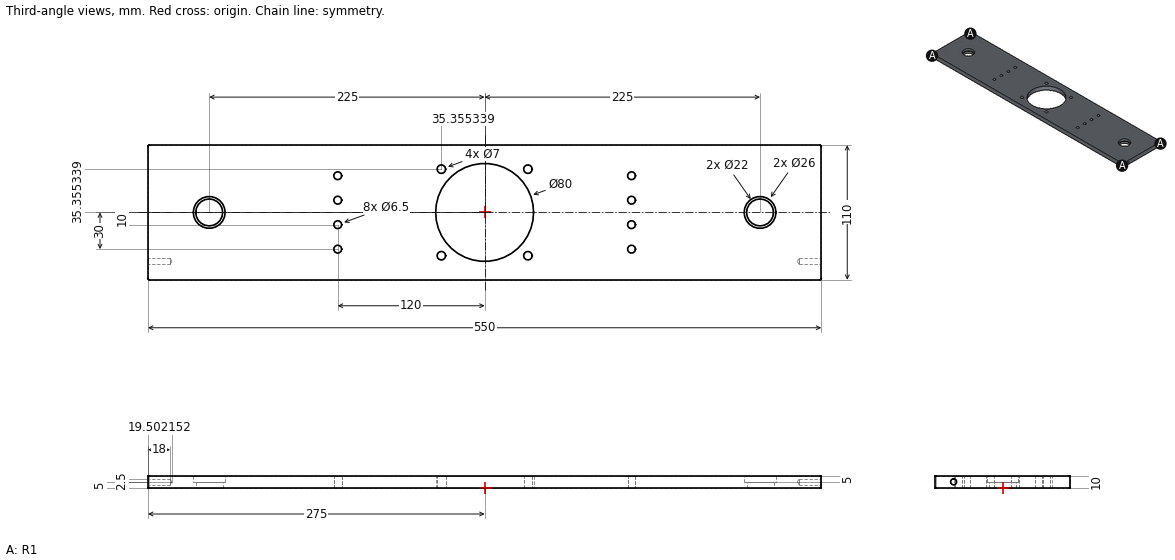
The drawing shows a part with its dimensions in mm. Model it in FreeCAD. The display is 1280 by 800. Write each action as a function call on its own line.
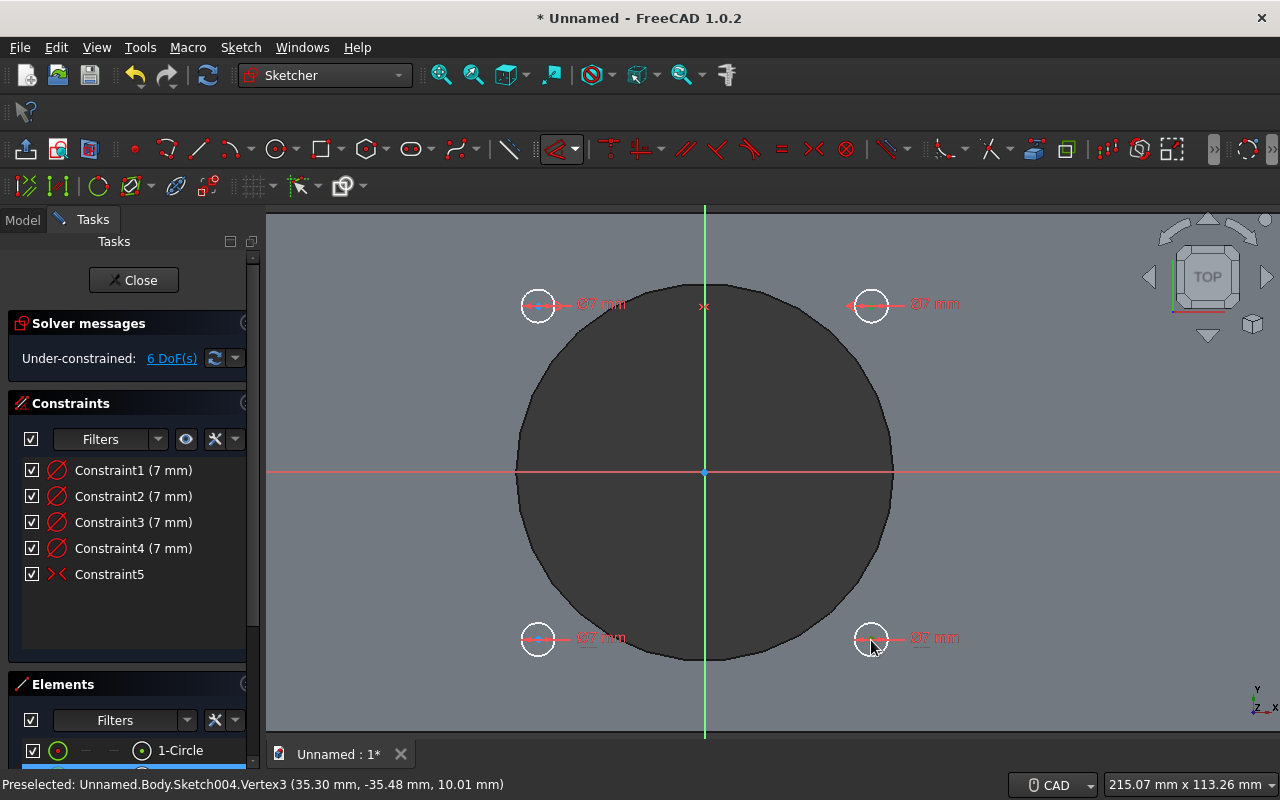
click(353, 472)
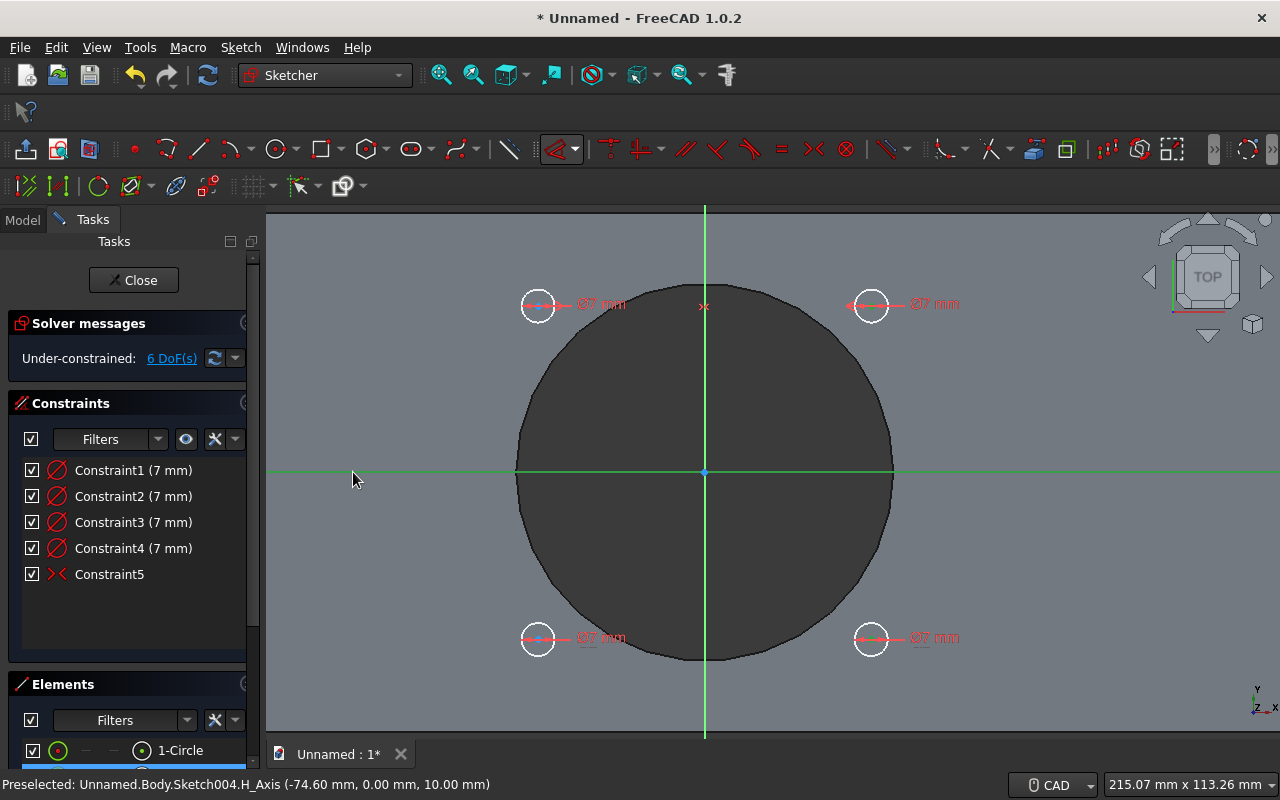
click(814, 150)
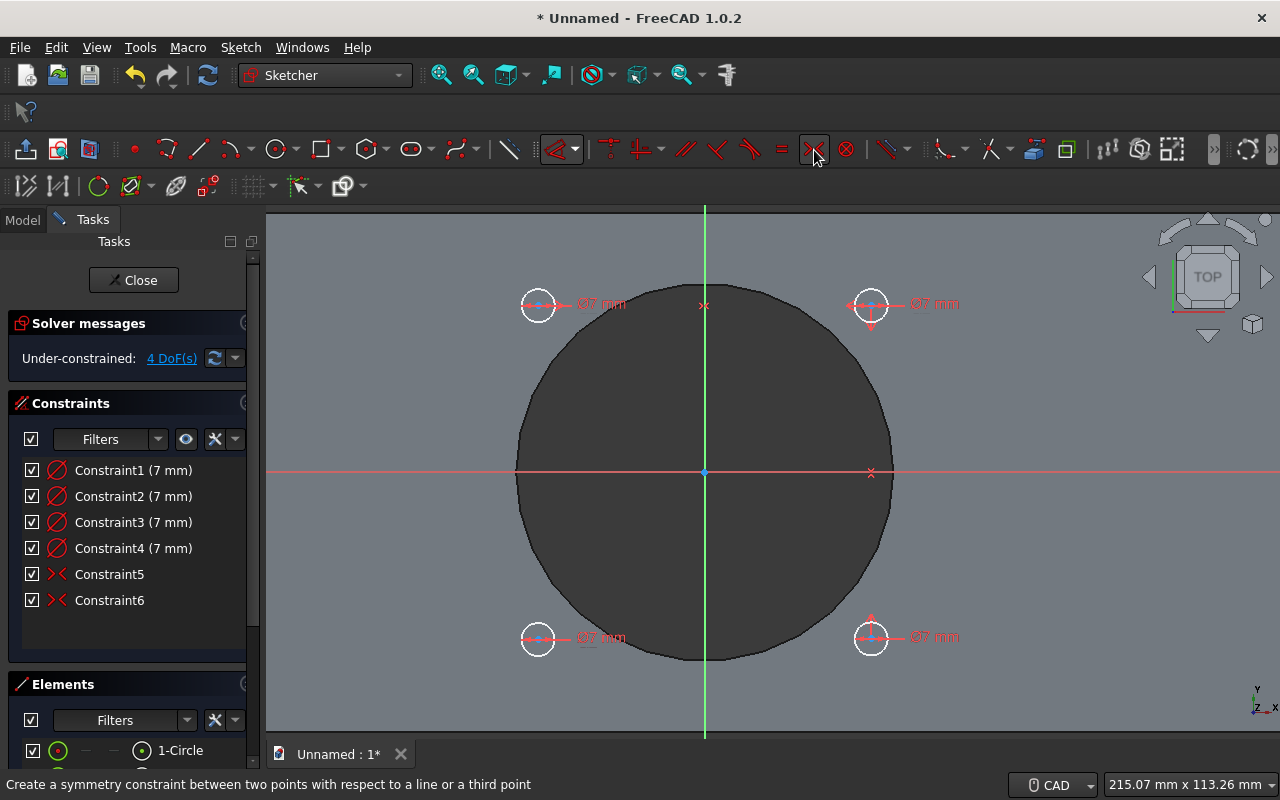
click(538, 306)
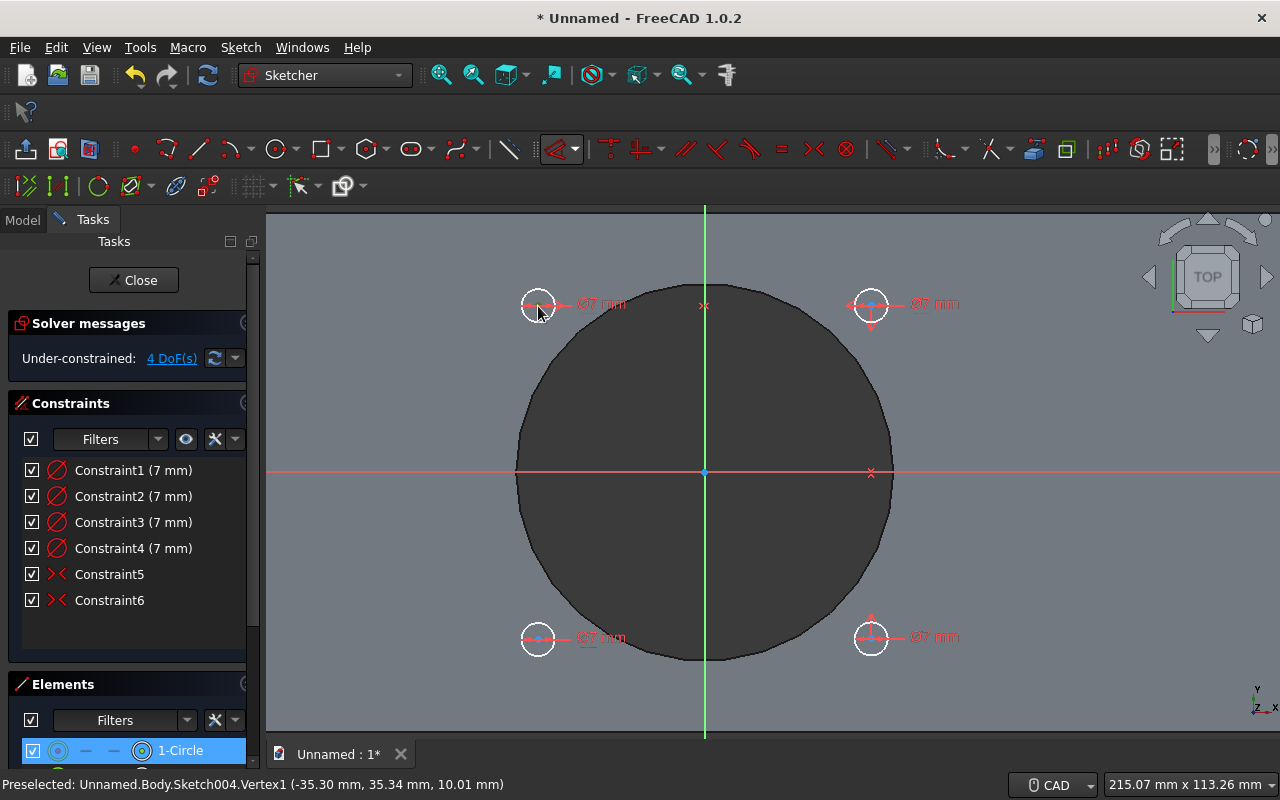
click(538, 640)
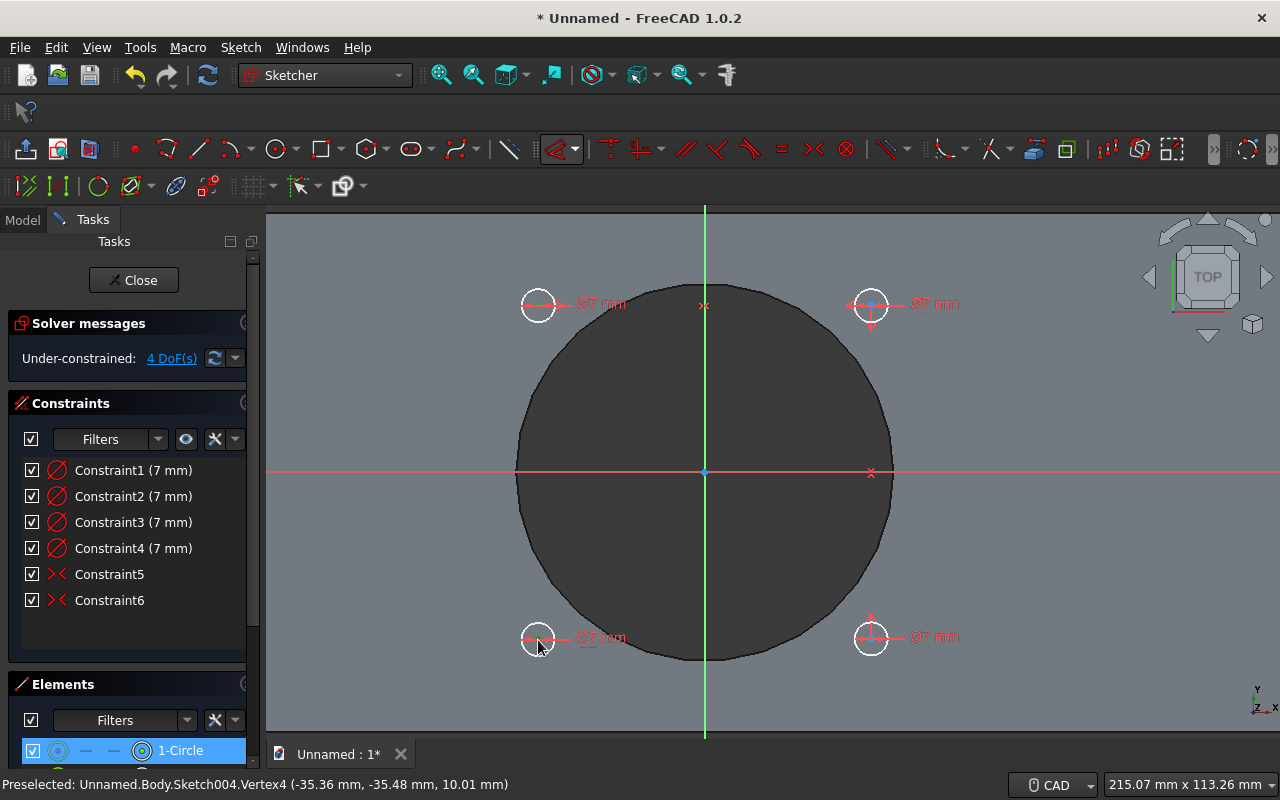
click(353, 472)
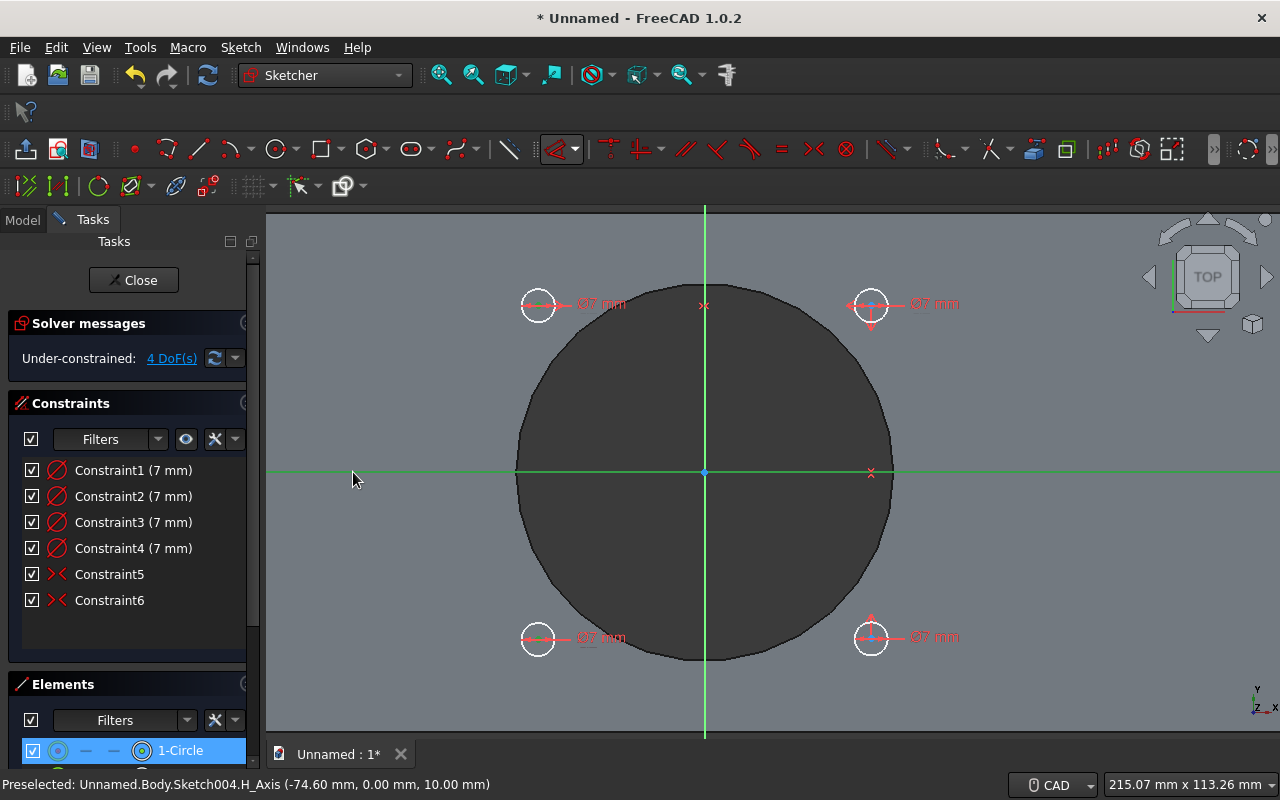
key(s)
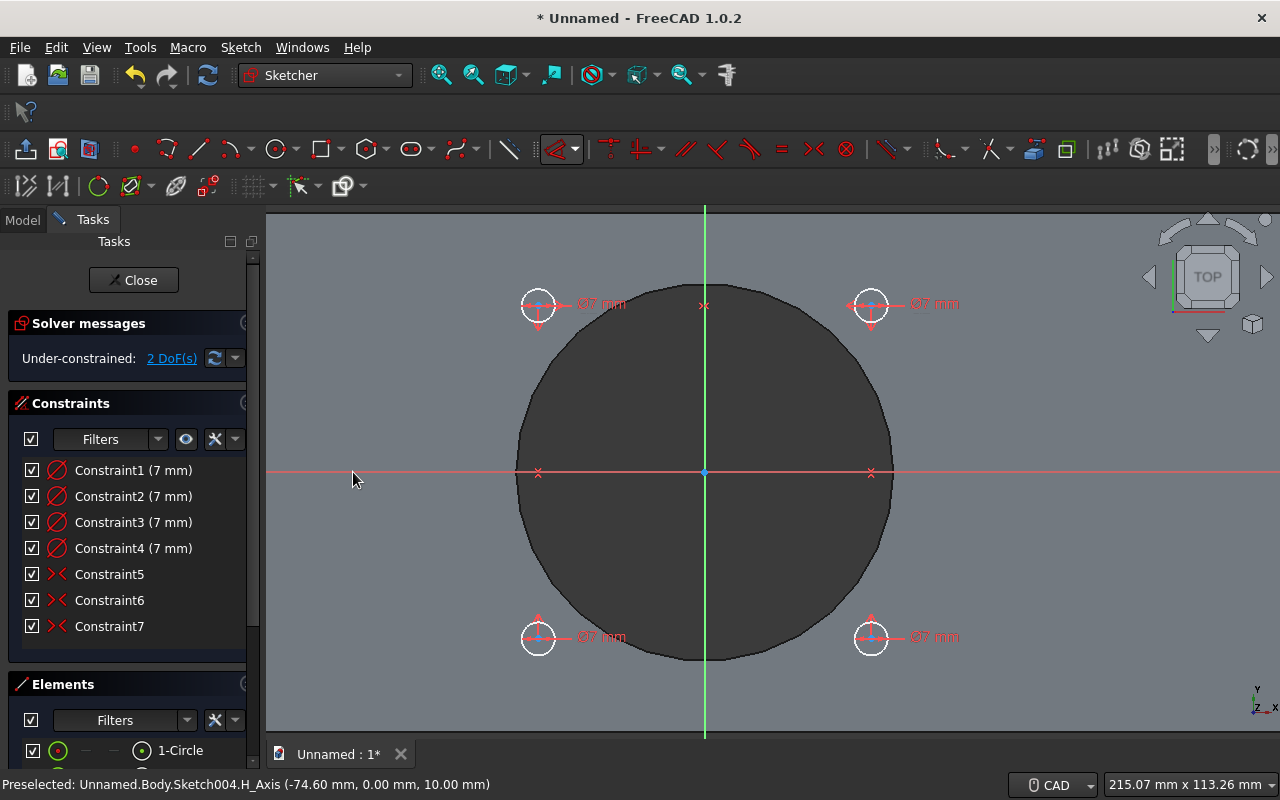
click(538, 306)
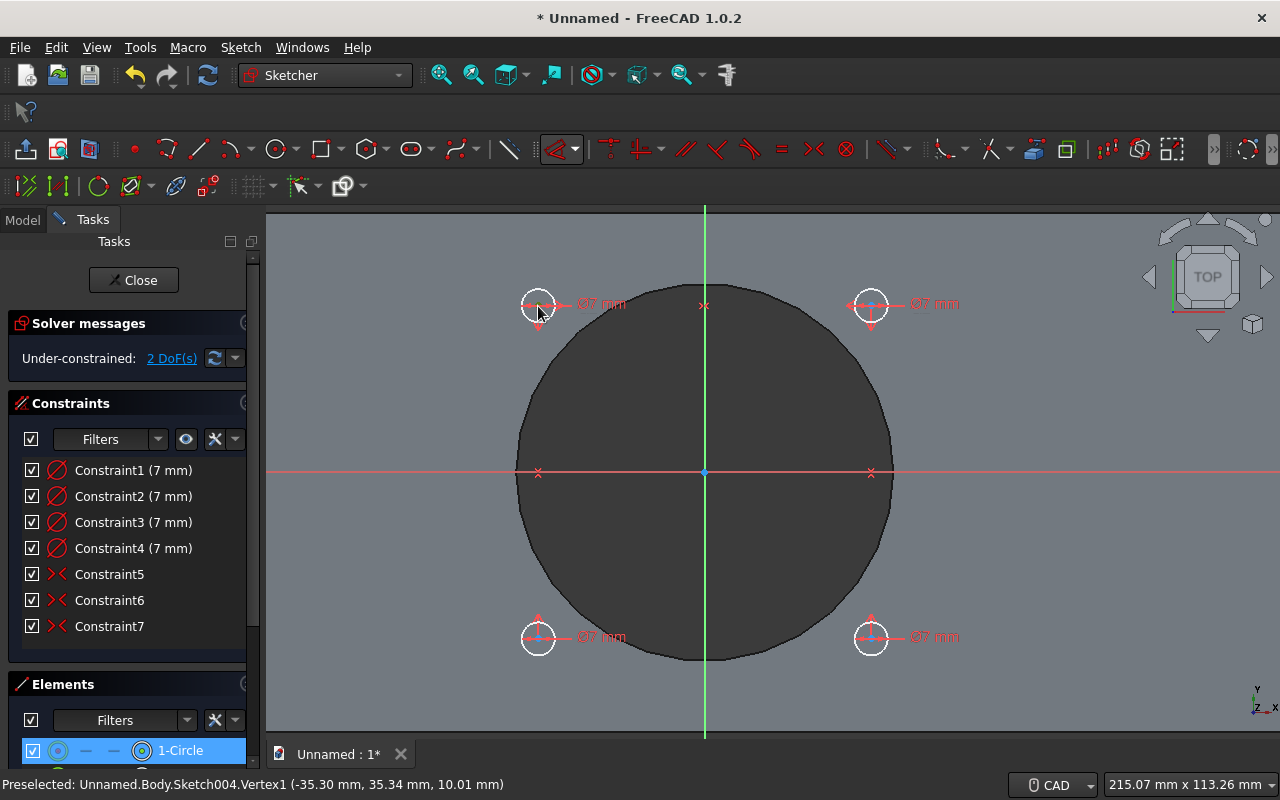
click(578, 150)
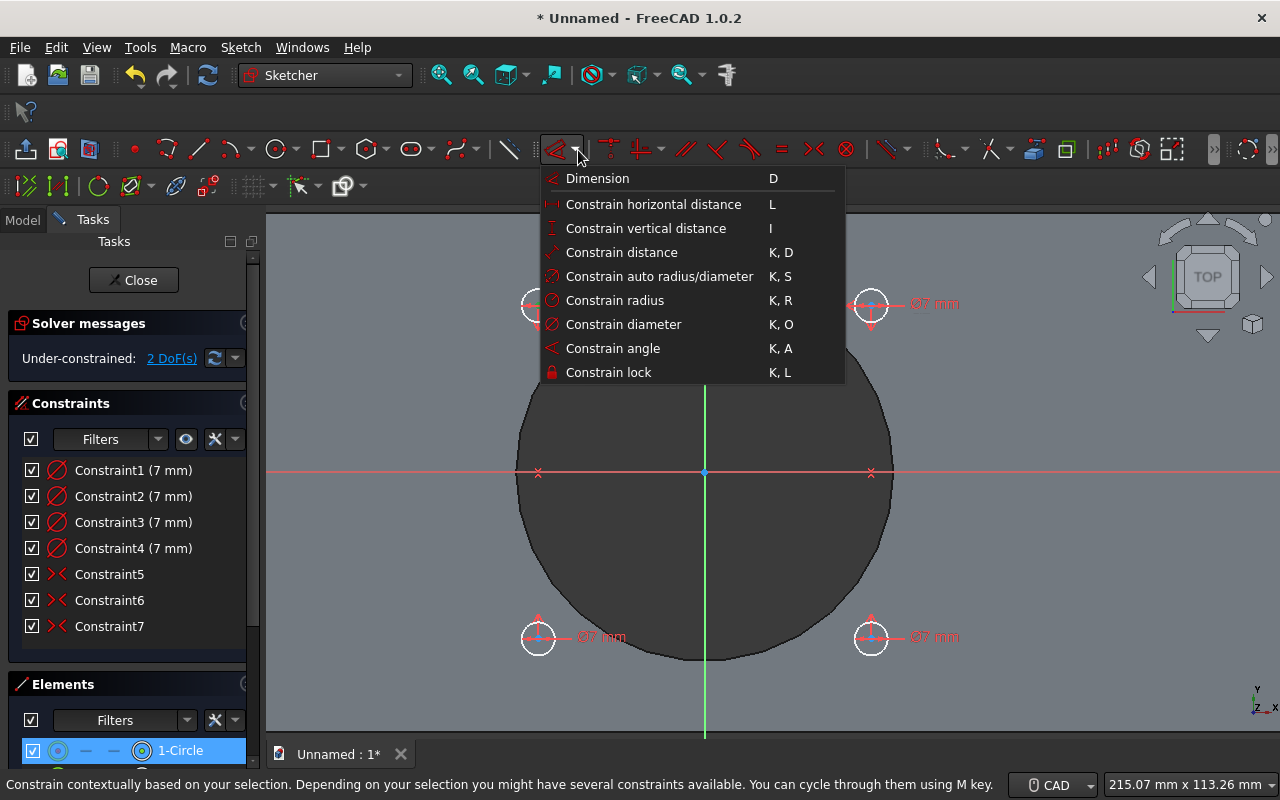
click(693, 204)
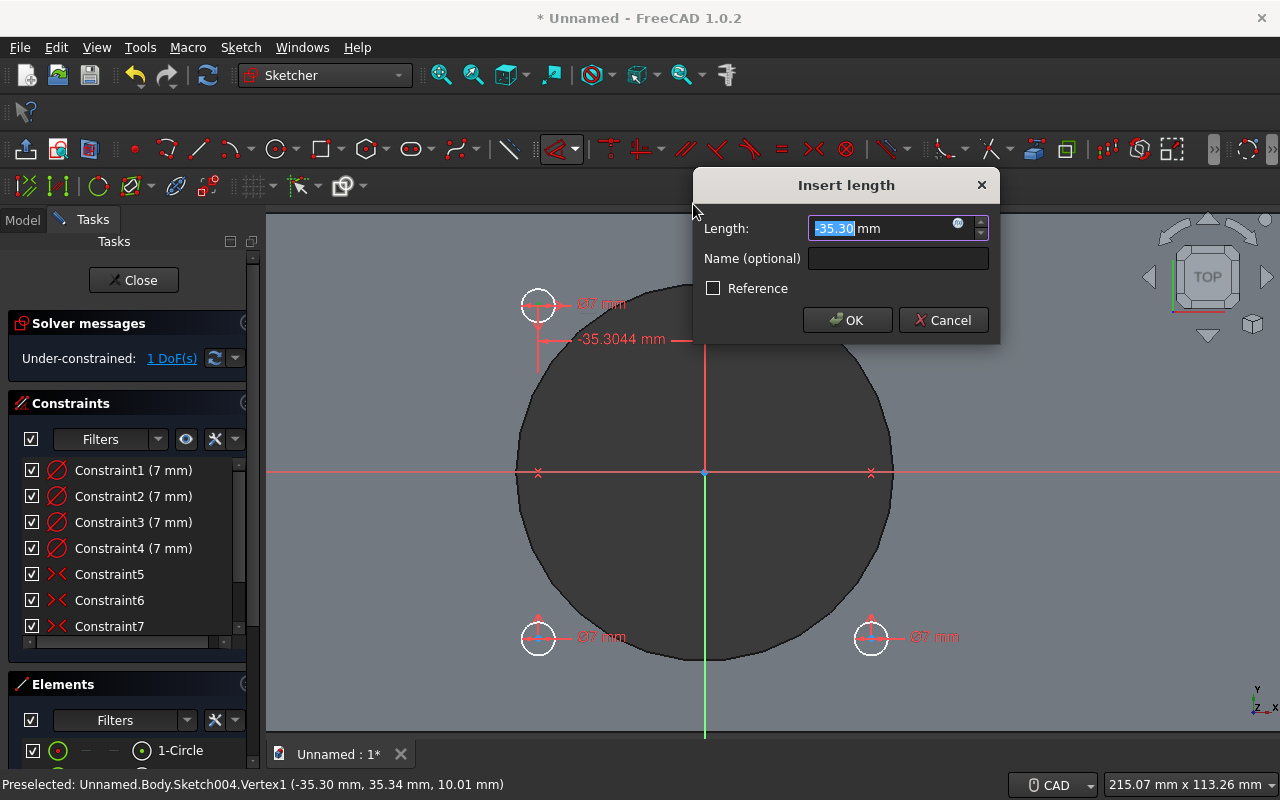
text(-35.355339)
key(Return)